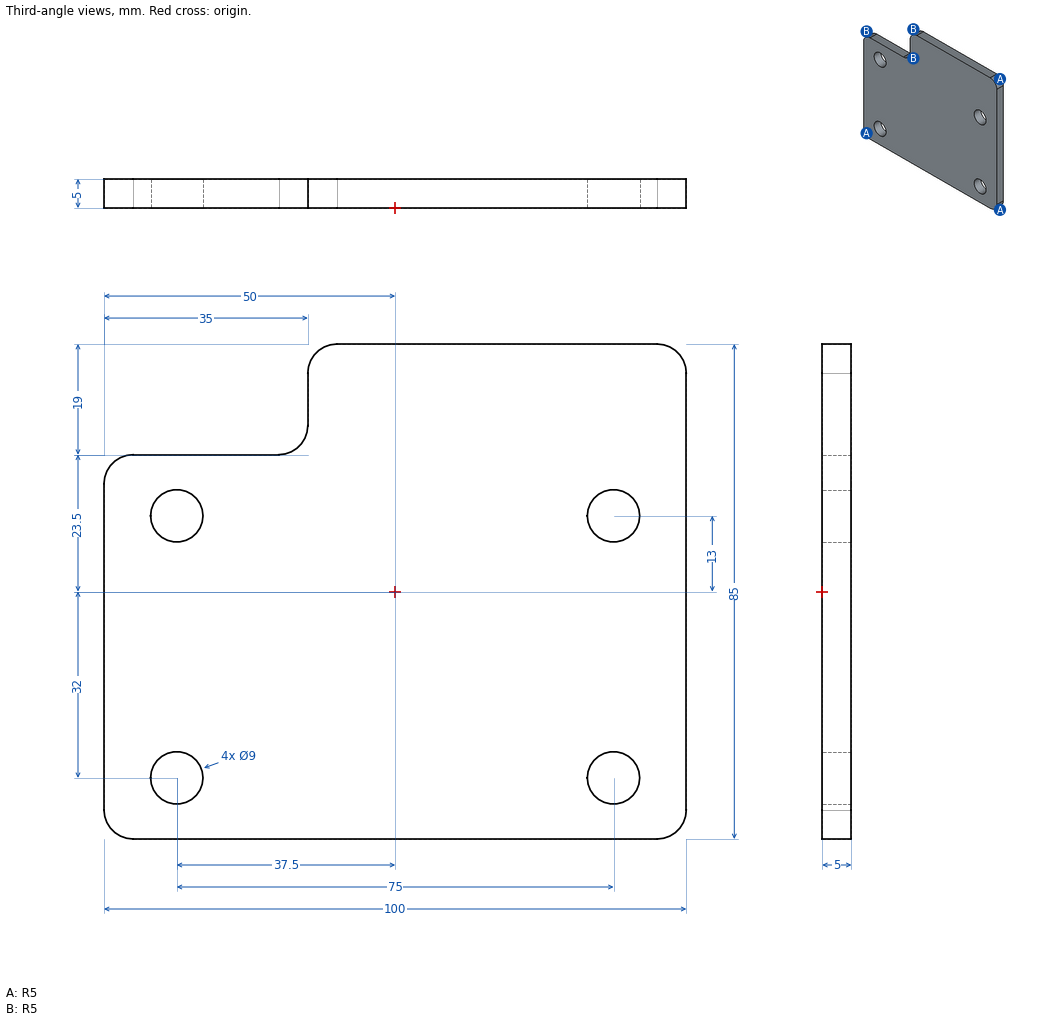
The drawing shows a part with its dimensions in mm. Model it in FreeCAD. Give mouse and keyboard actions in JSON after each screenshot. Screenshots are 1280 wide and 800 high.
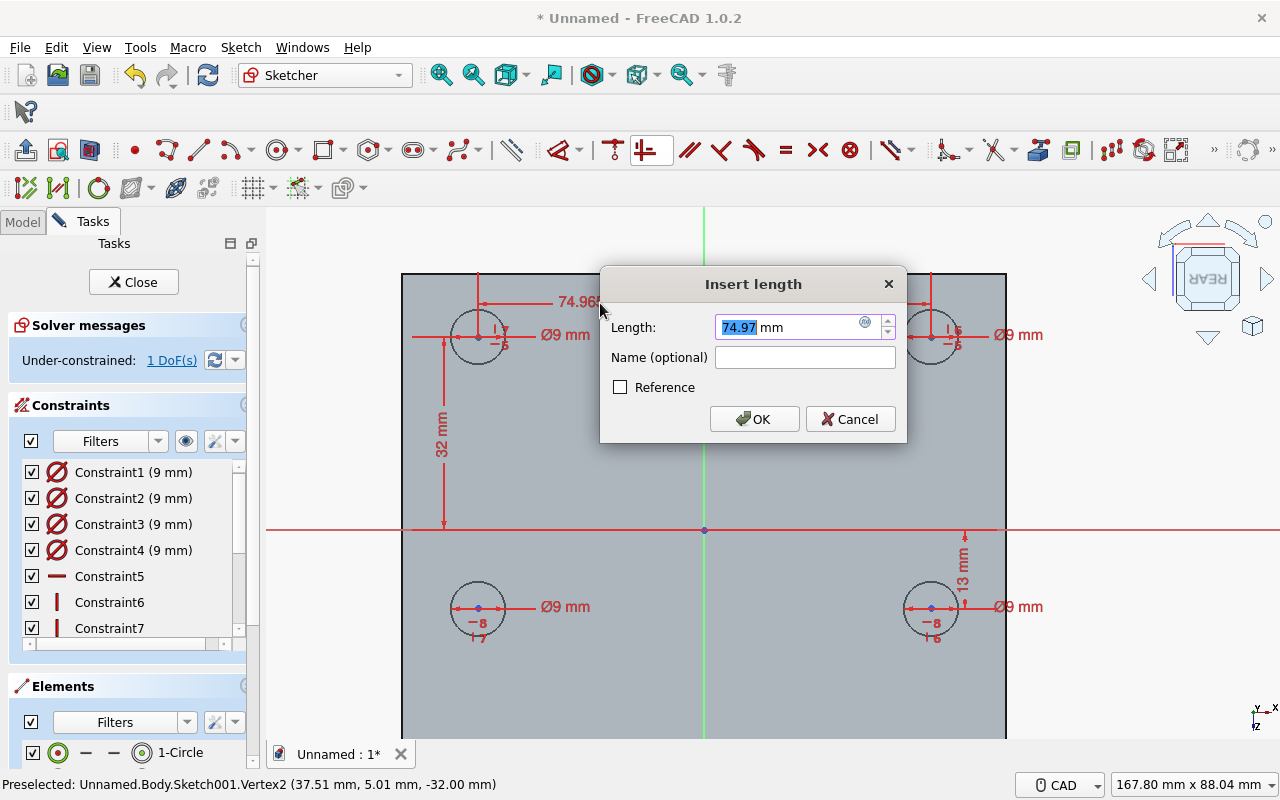
{"action": "type", "text": "75"}
{"action": "key", "text": "Return"}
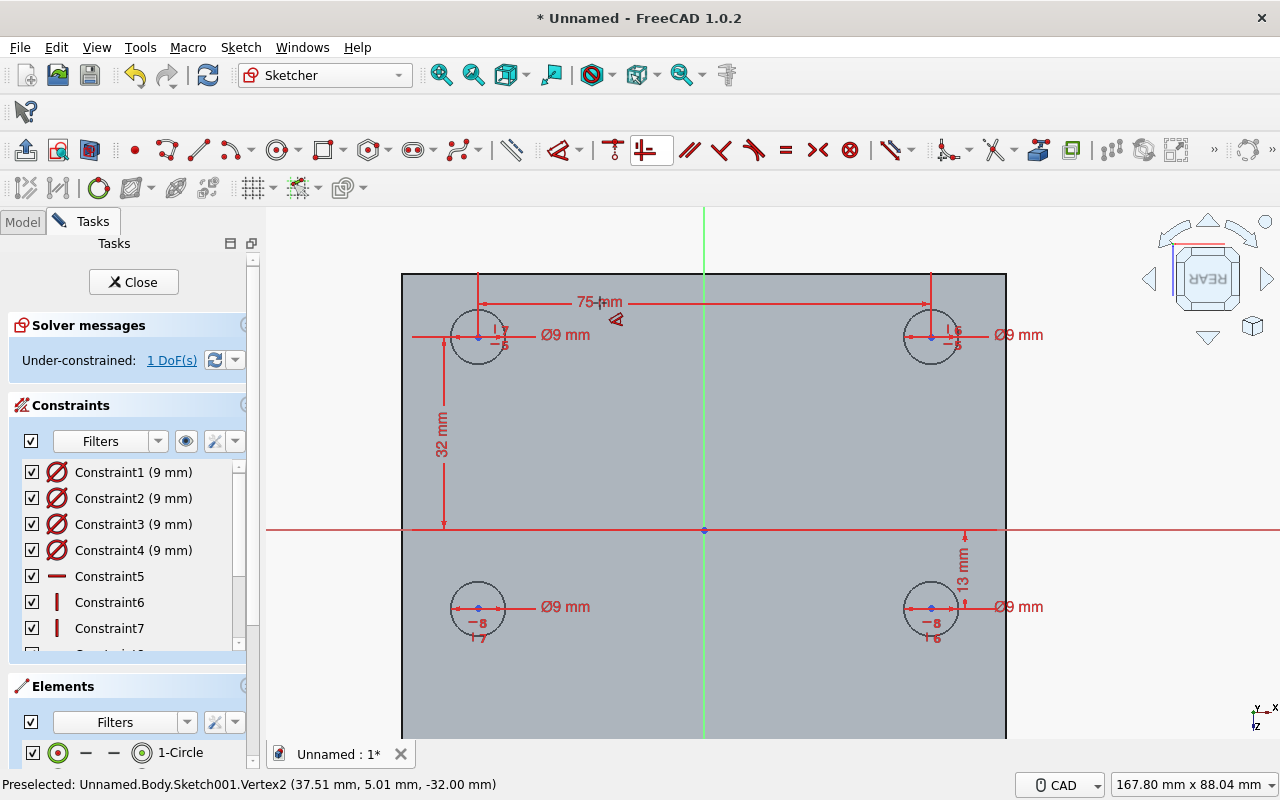
{"action": "left_click", "coordinate": [478, 337]}
{"action": "left_click", "coordinate": [512, 303]}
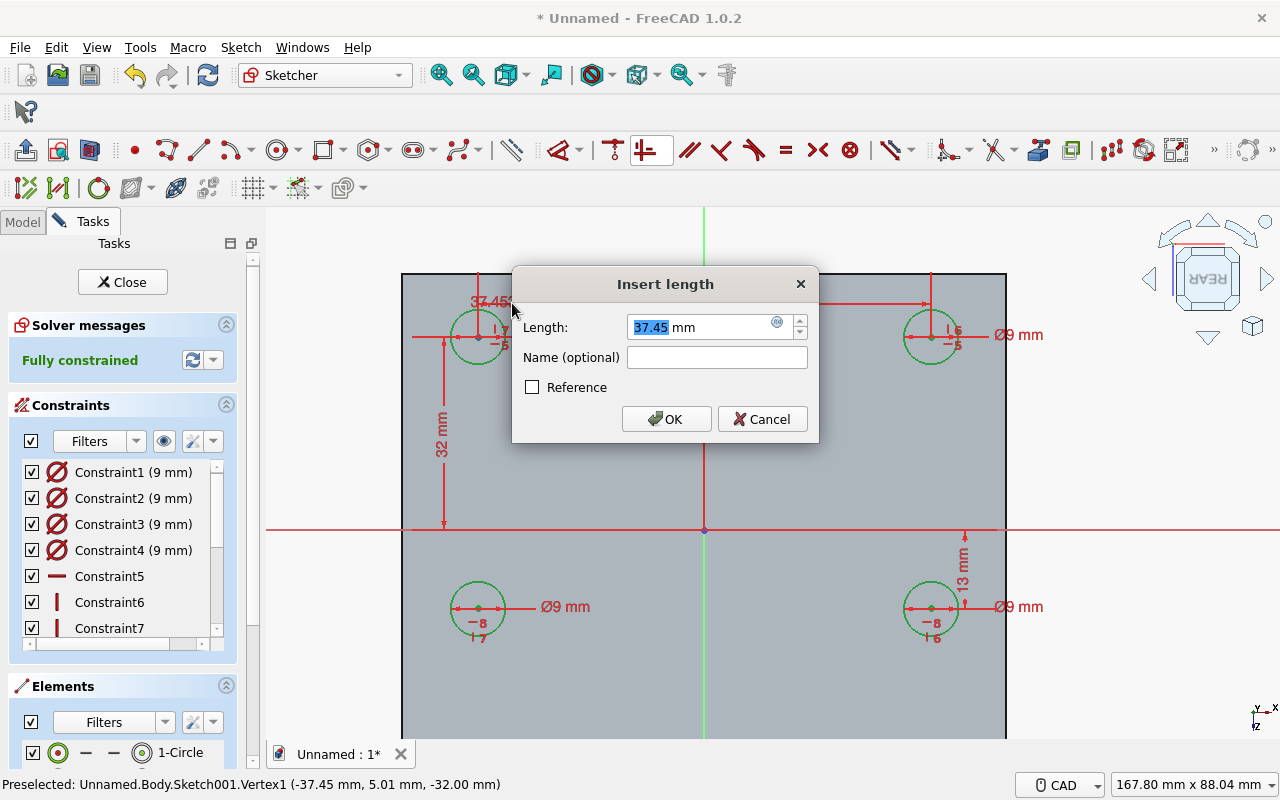
{"action": "type", "text": "37.5"}
{"action": "key", "text": "Return"}
{"action": "key", "text": "Escape"}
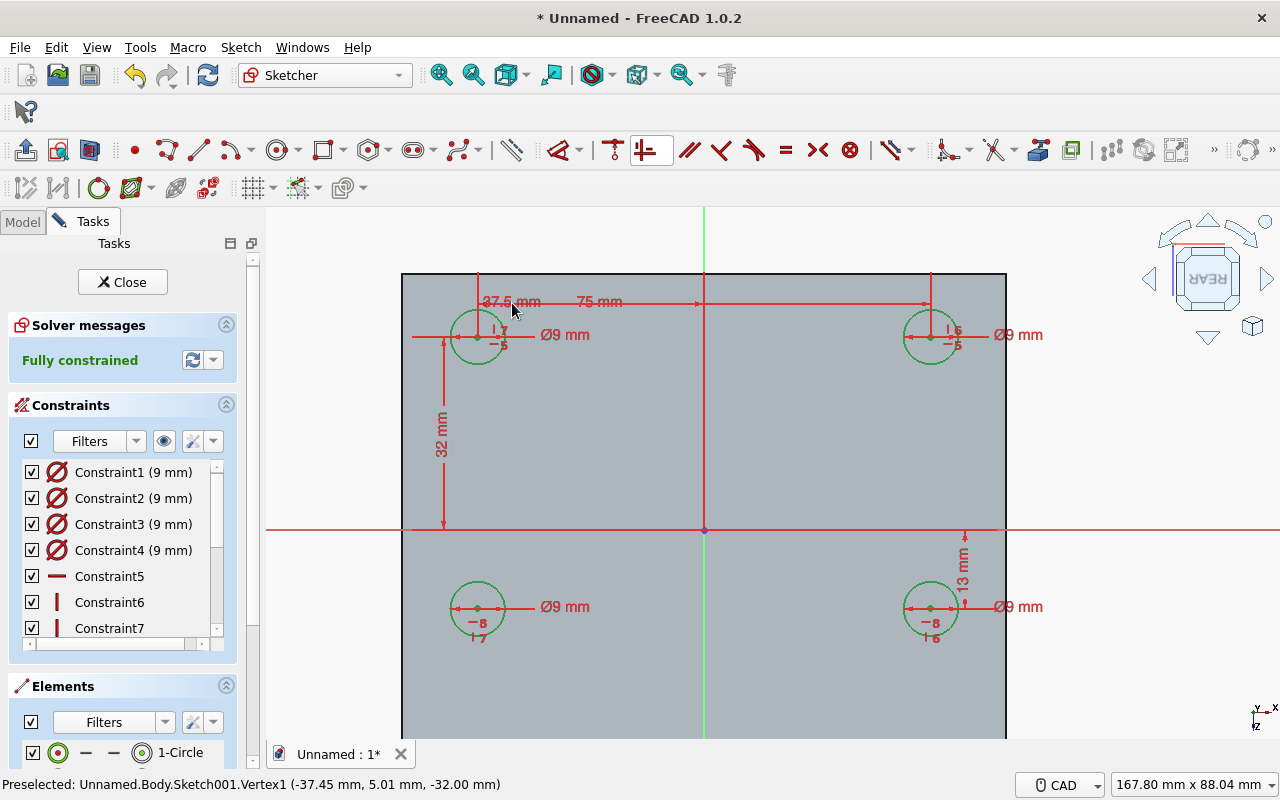
{"action": "left_click", "coordinate": [123, 282]}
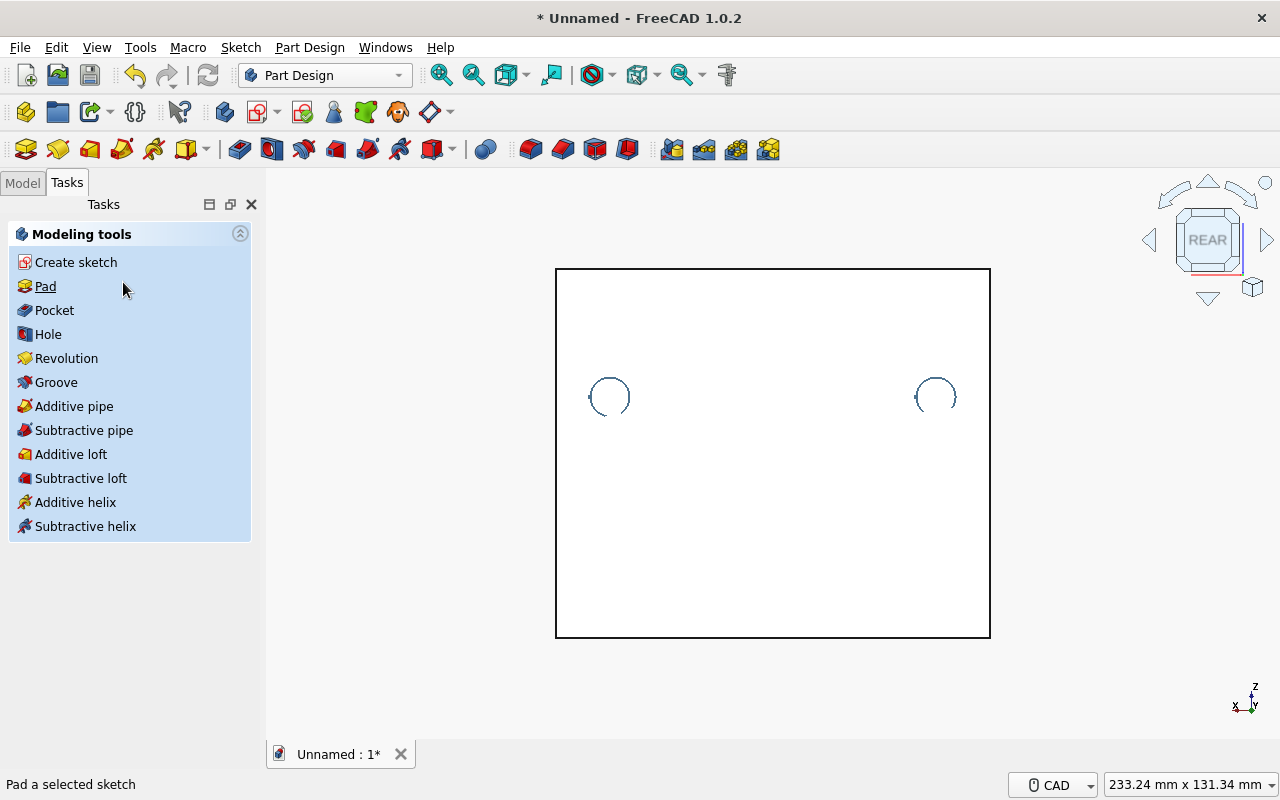
{"action": "left_click", "coordinate": [240, 150]}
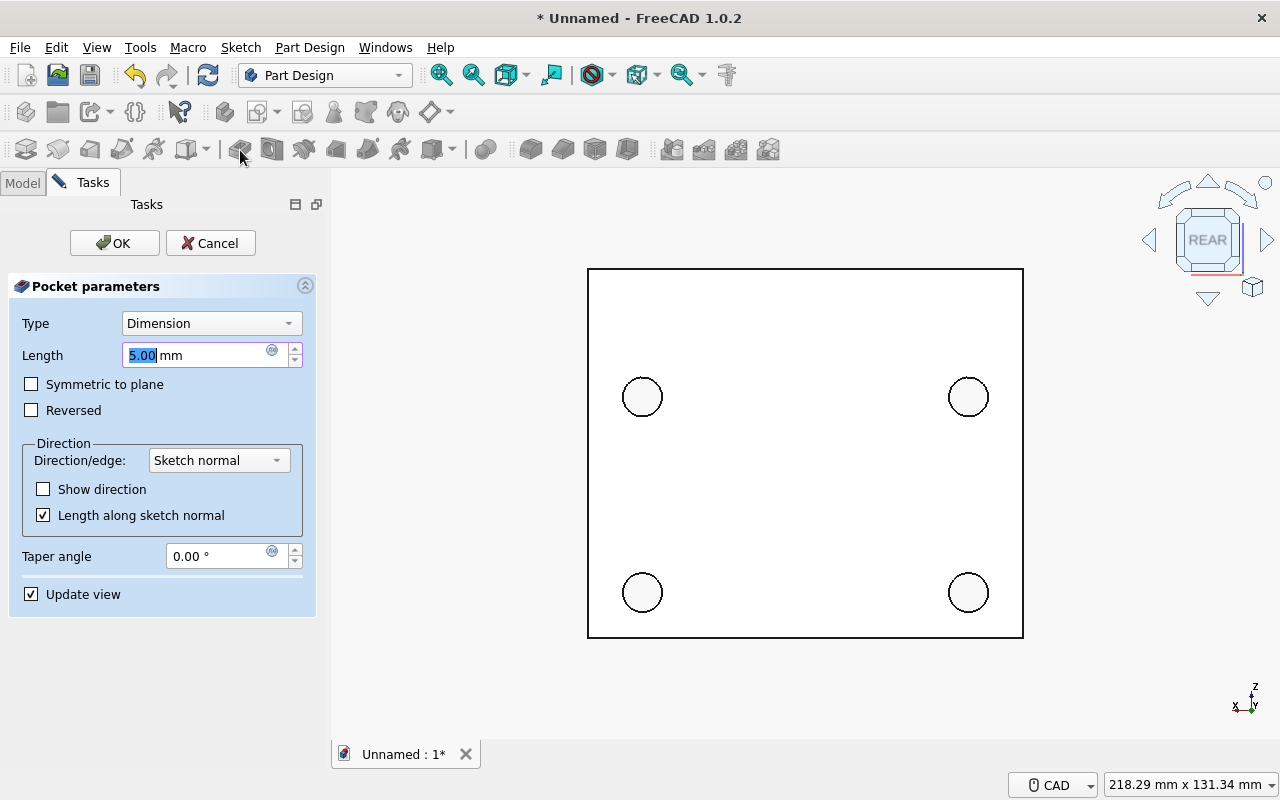
{"action": "left_click", "coordinate": [212, 324]}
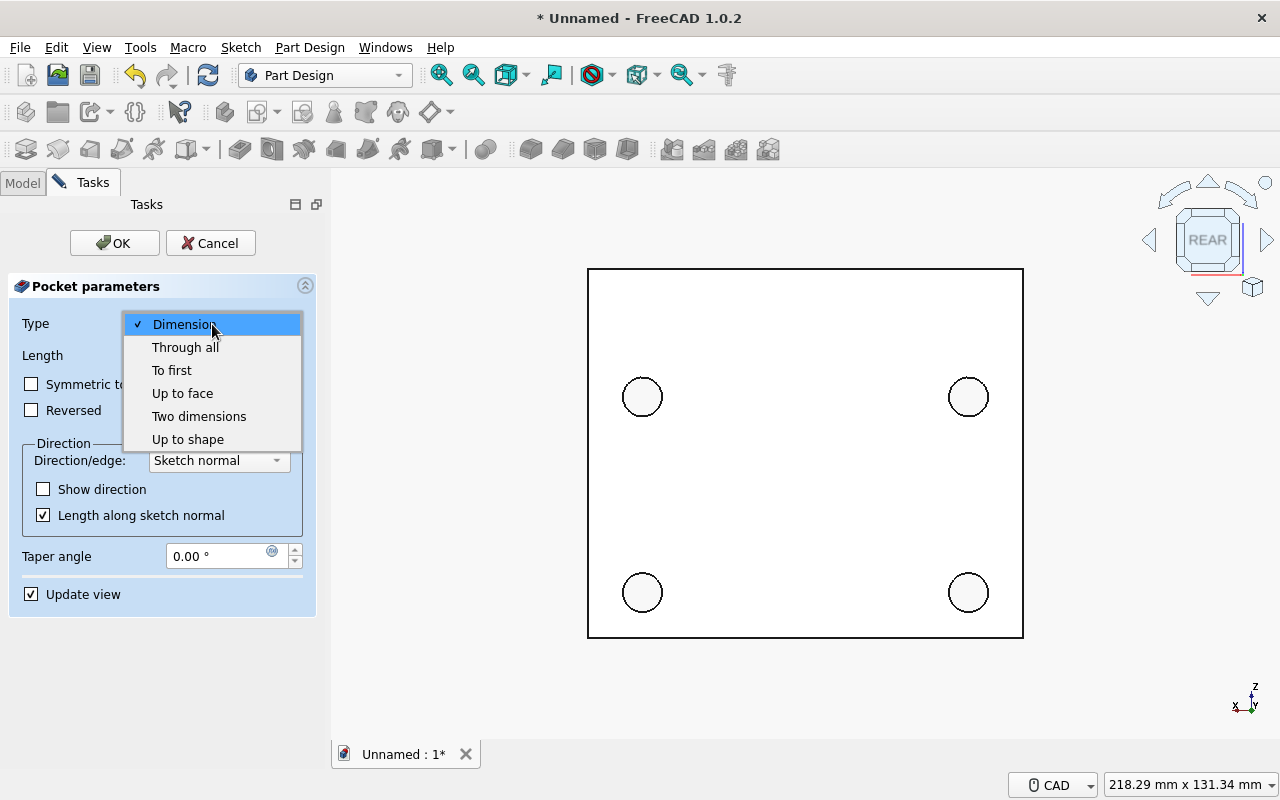
{"action": "left_click", "coordinate": [212, 348]}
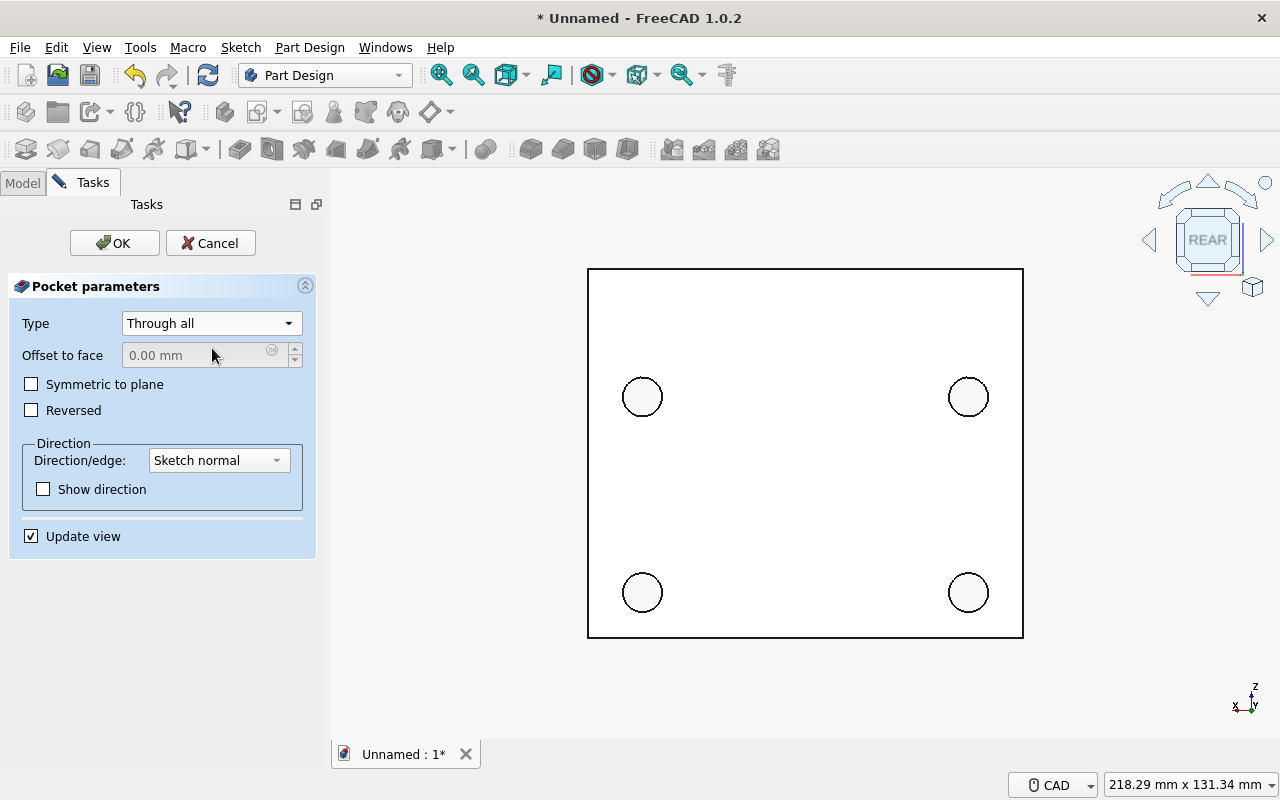
{"action": "left_click", "coordinate": [115, 243]}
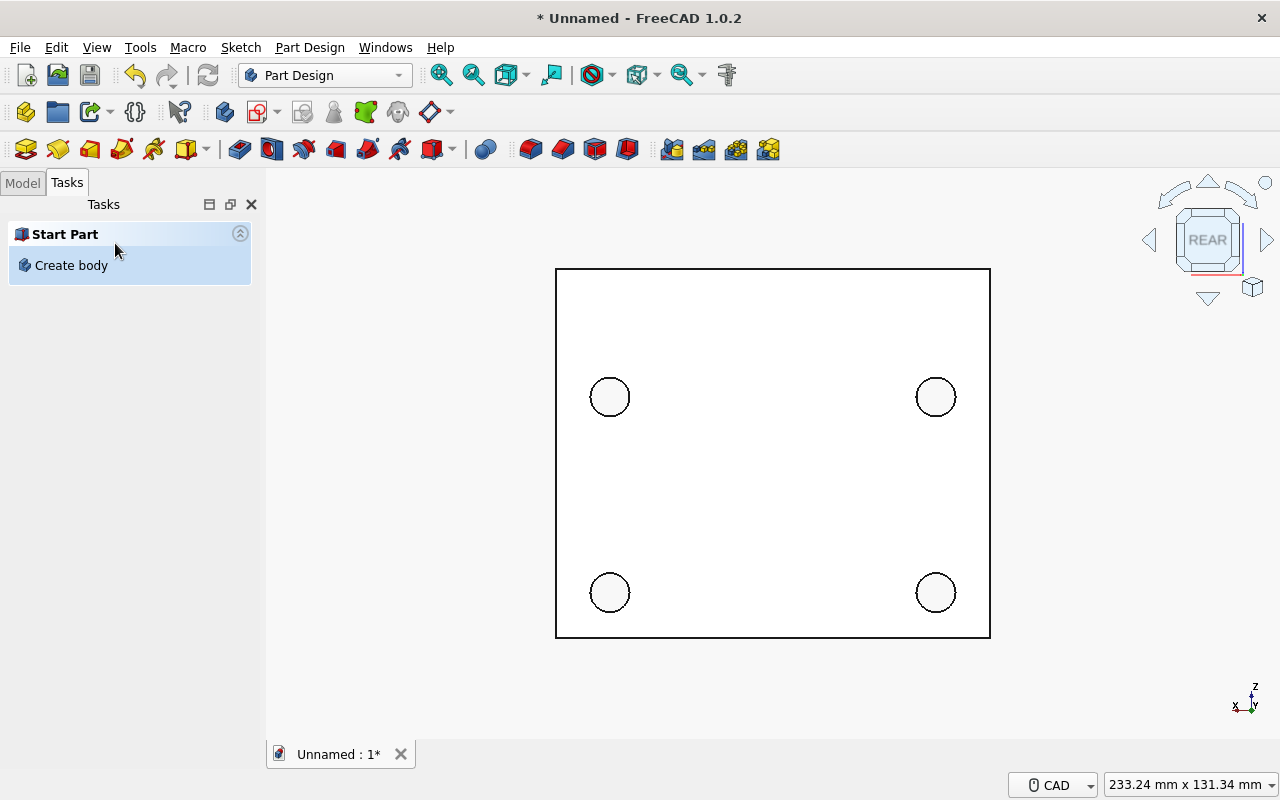
{"action": "scroll", "coordinate": [556, 268], "scroll_direction": "up", "scroll_amount": 4}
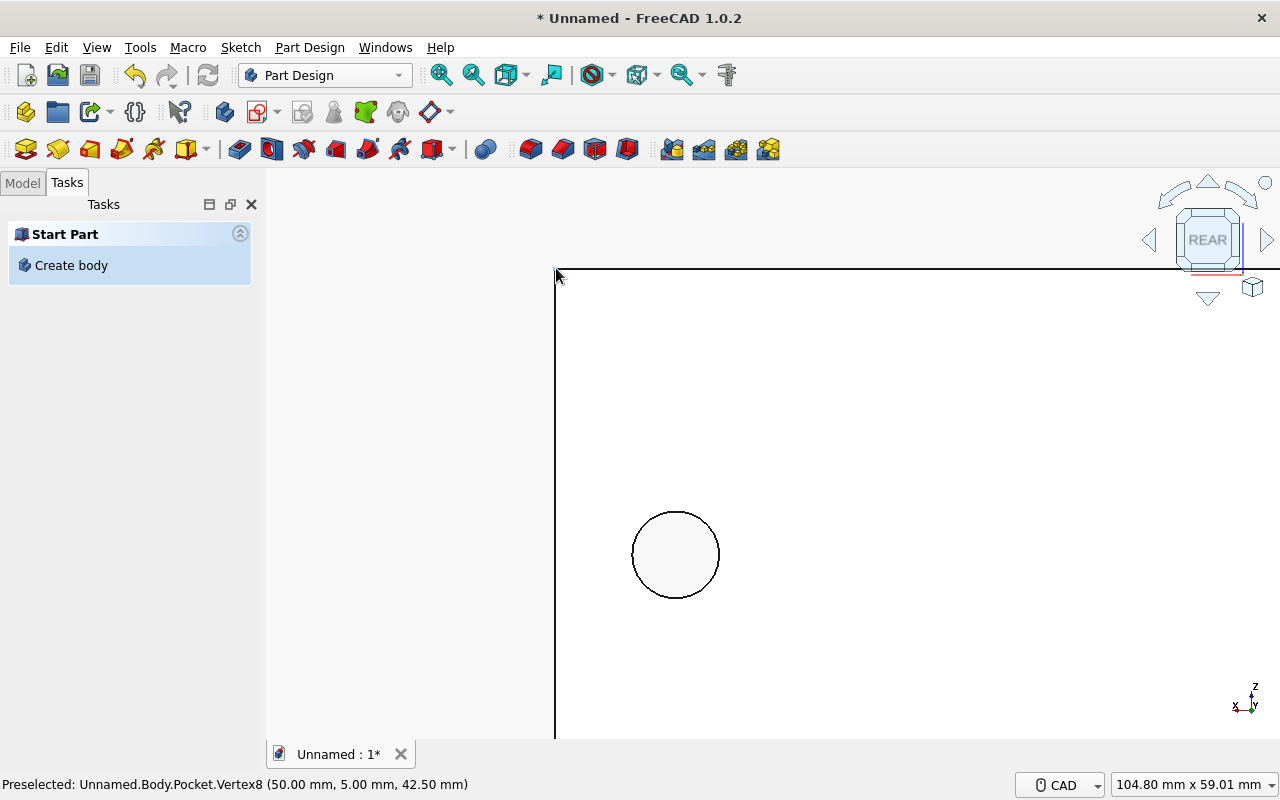
{"action": "key", "text": "v f"}